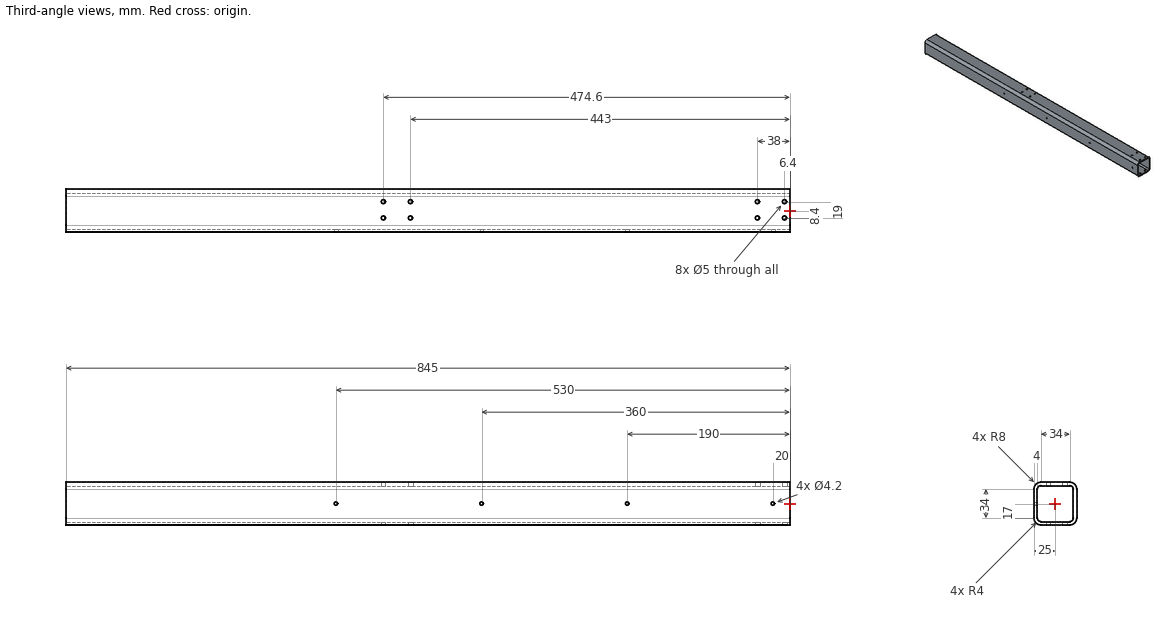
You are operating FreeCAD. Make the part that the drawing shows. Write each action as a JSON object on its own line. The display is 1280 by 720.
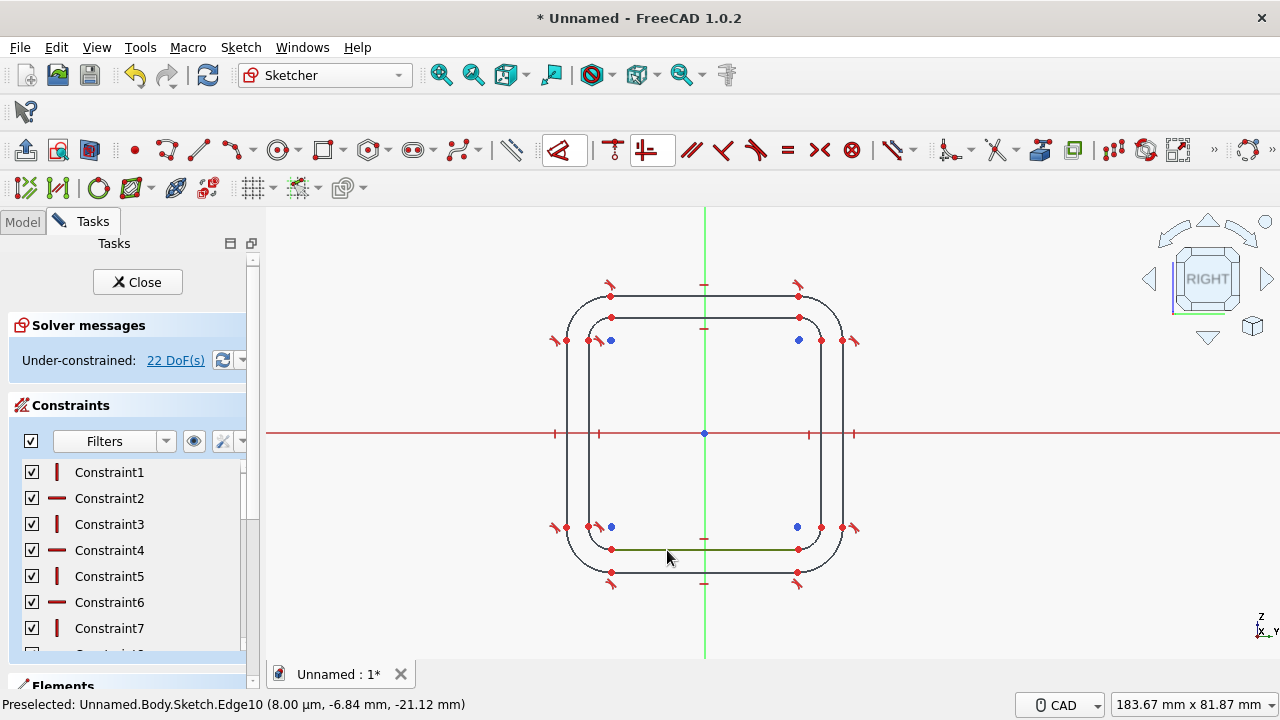
{"action": "scroll", "coordinate": [591, 537], "scroll_direction": "up", "scroll_amount": 2}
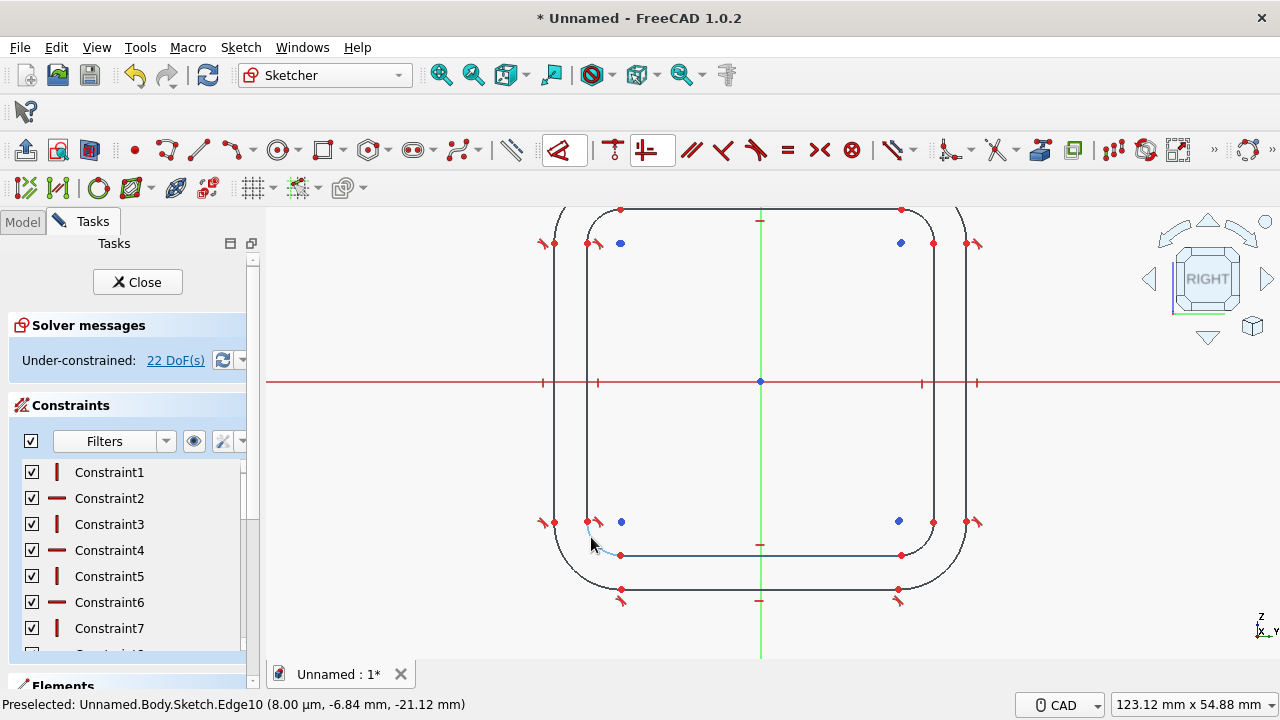
{"action": "left_click", "coordinate": [591, 537]}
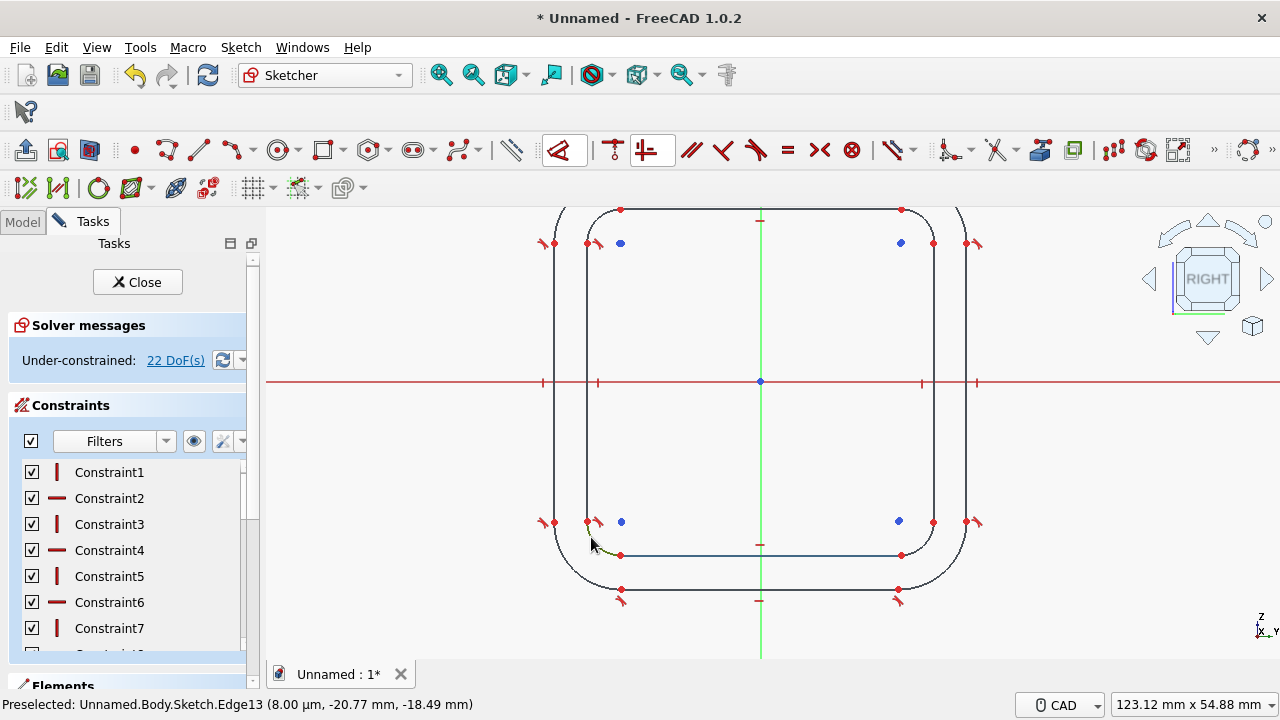
{"action": "left_click", "coordinate": [756, 150]}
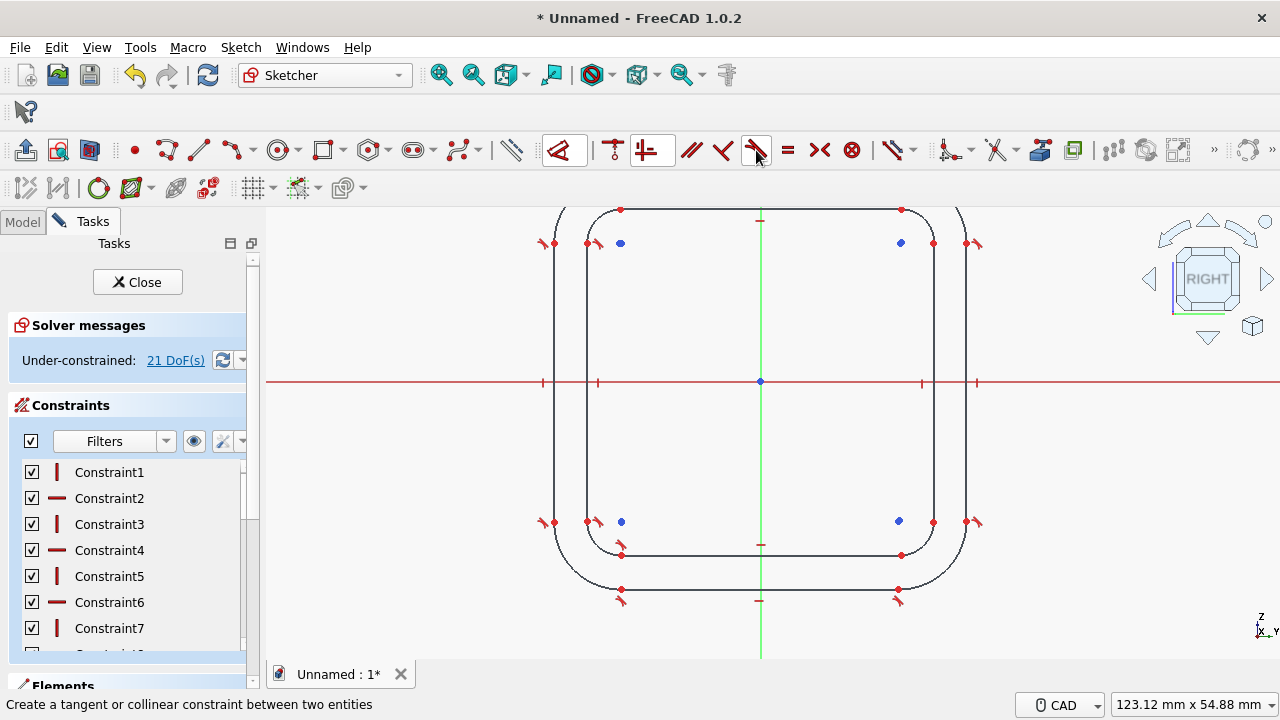
{"action": "left_click", "coordinate": [705, 556]}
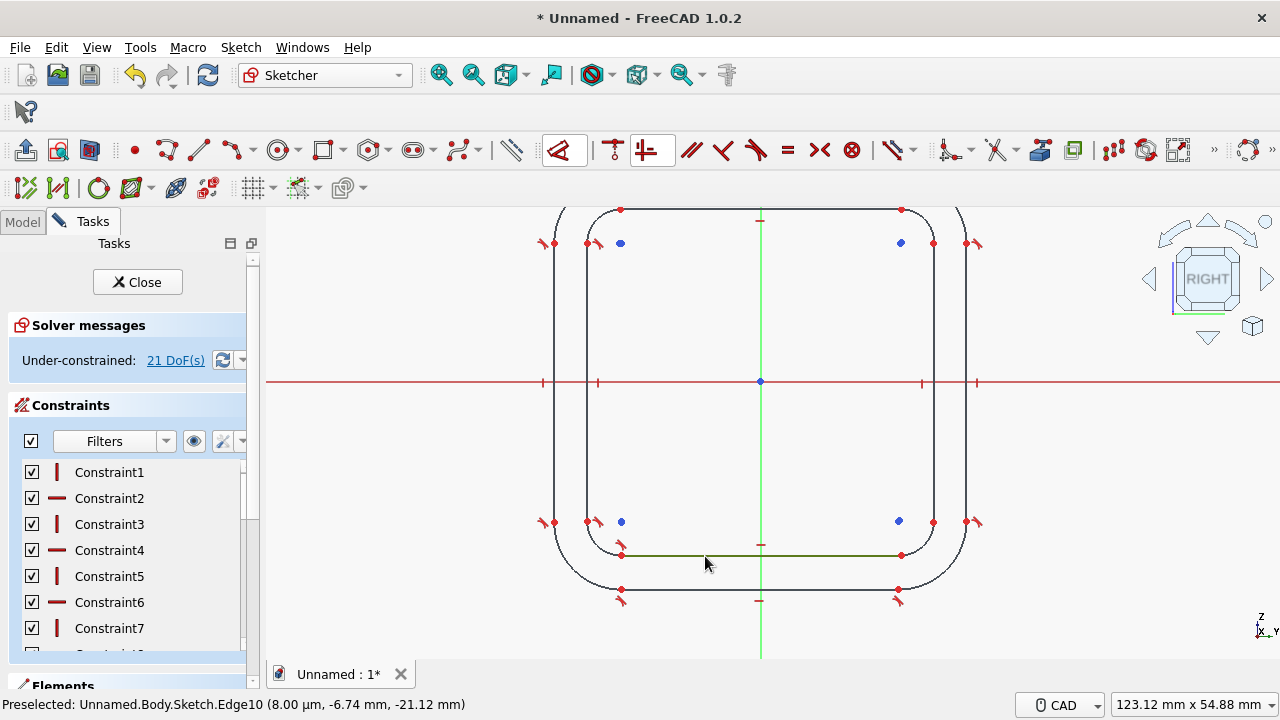
{"action": "left_click", "coordinate": [916, 551]}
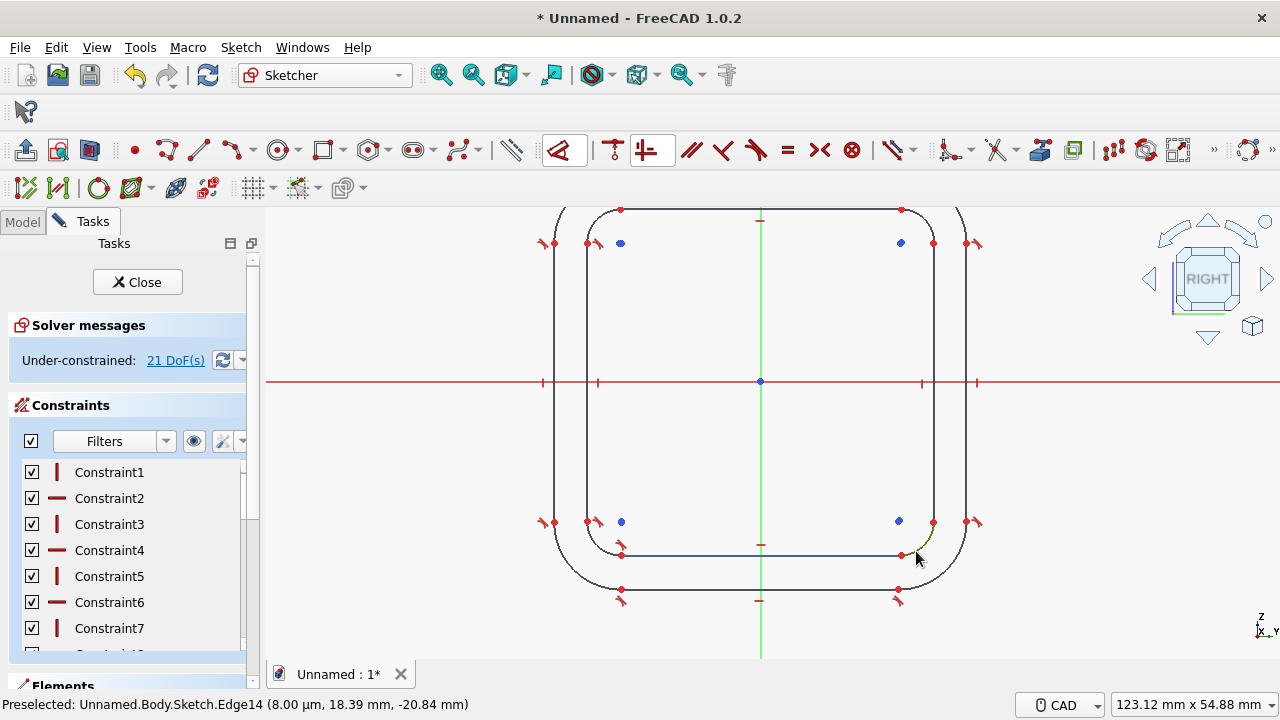
{"action": "left_click", "coordinate": [756, 150]}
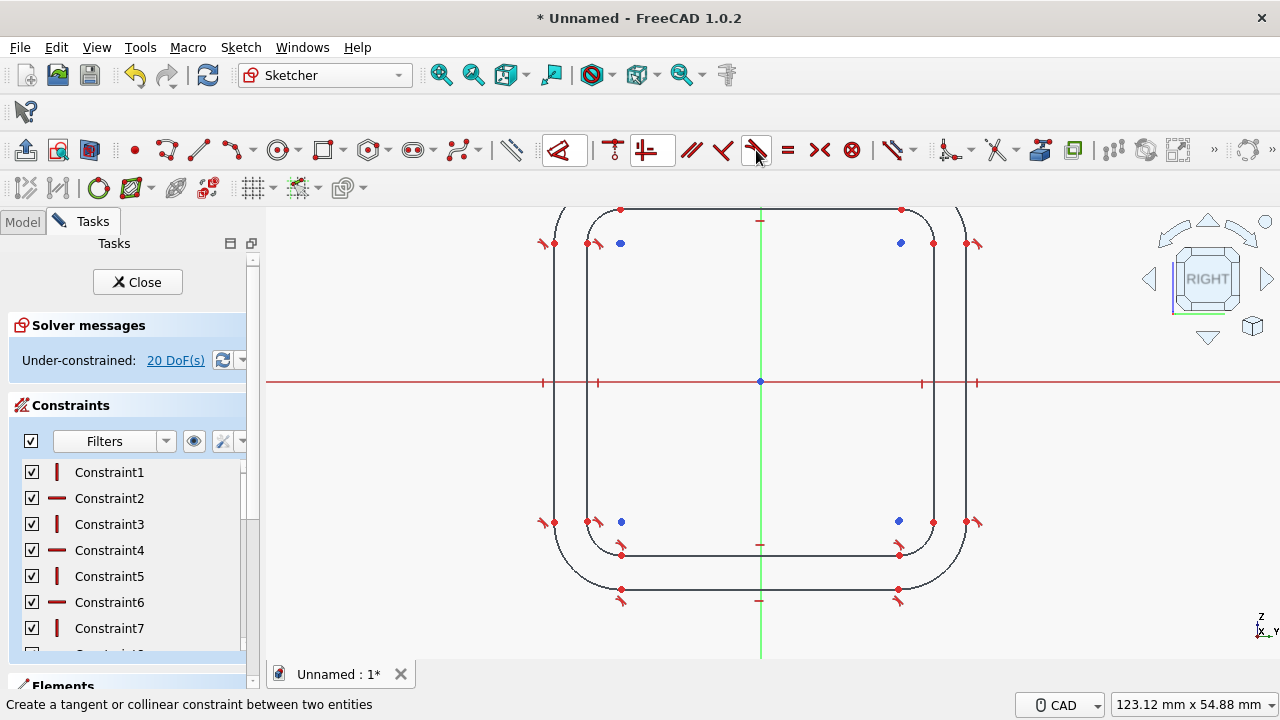
{"action": "left_click", "coordinate": [934, 439]}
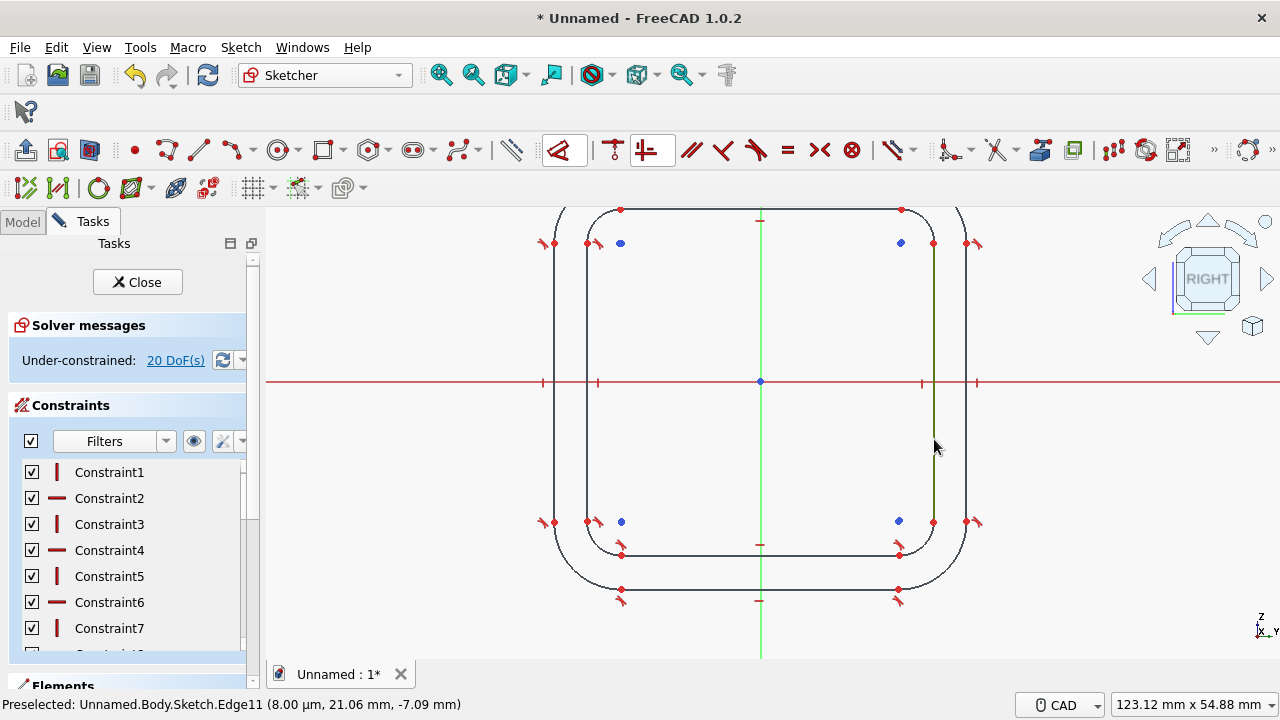
{"action": "left_click", "coordinate": [915, 552]}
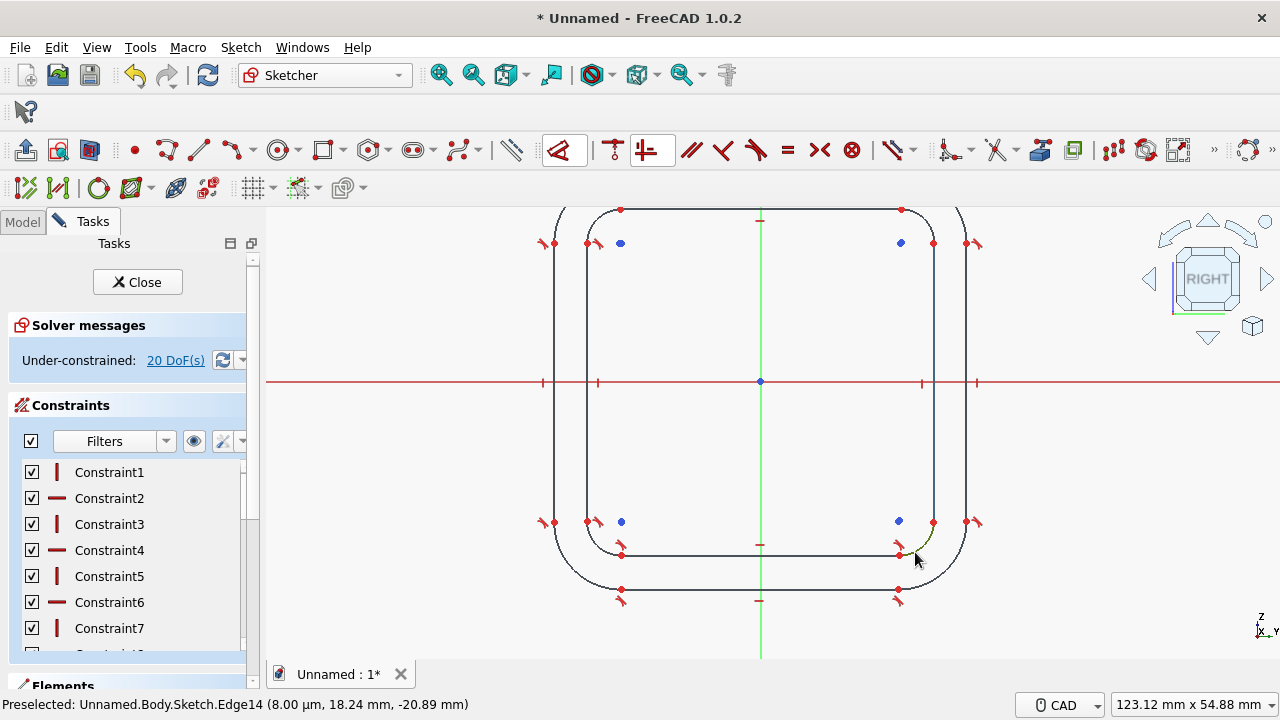
{"action": "left_click", "coordinate": [756, 150]}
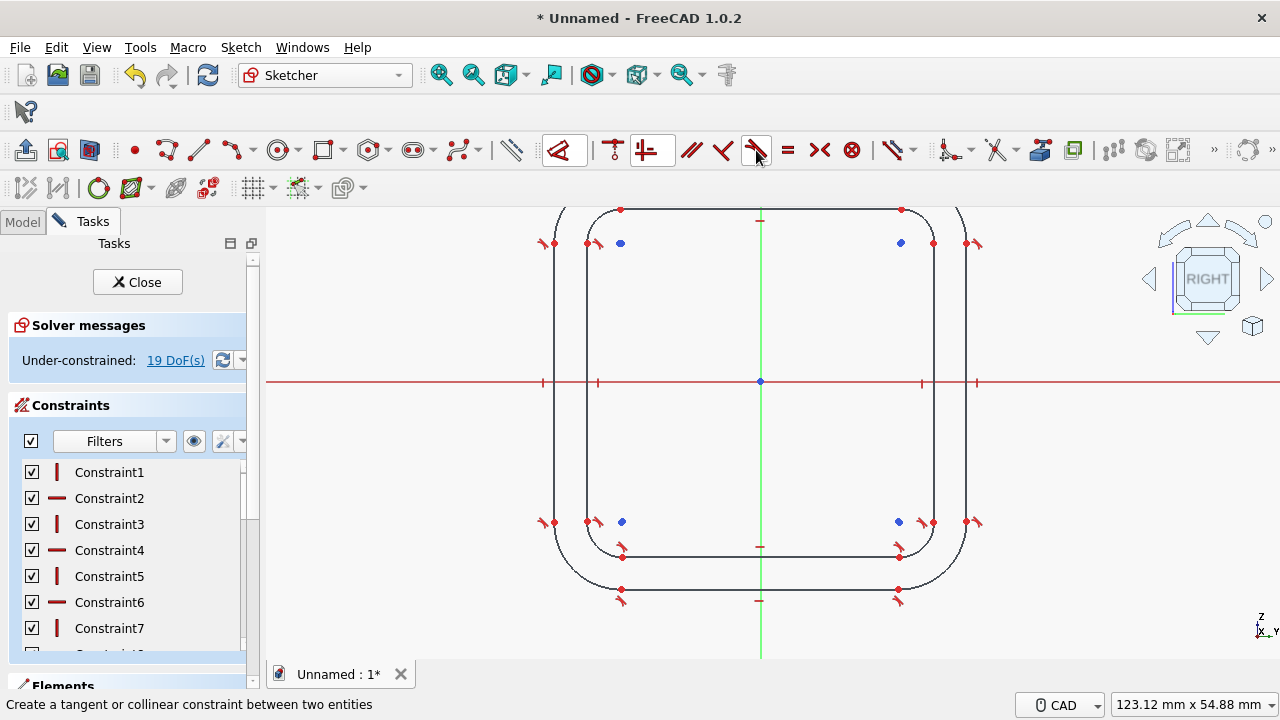
{"action": "left_click", "coordinate": [934, 439]}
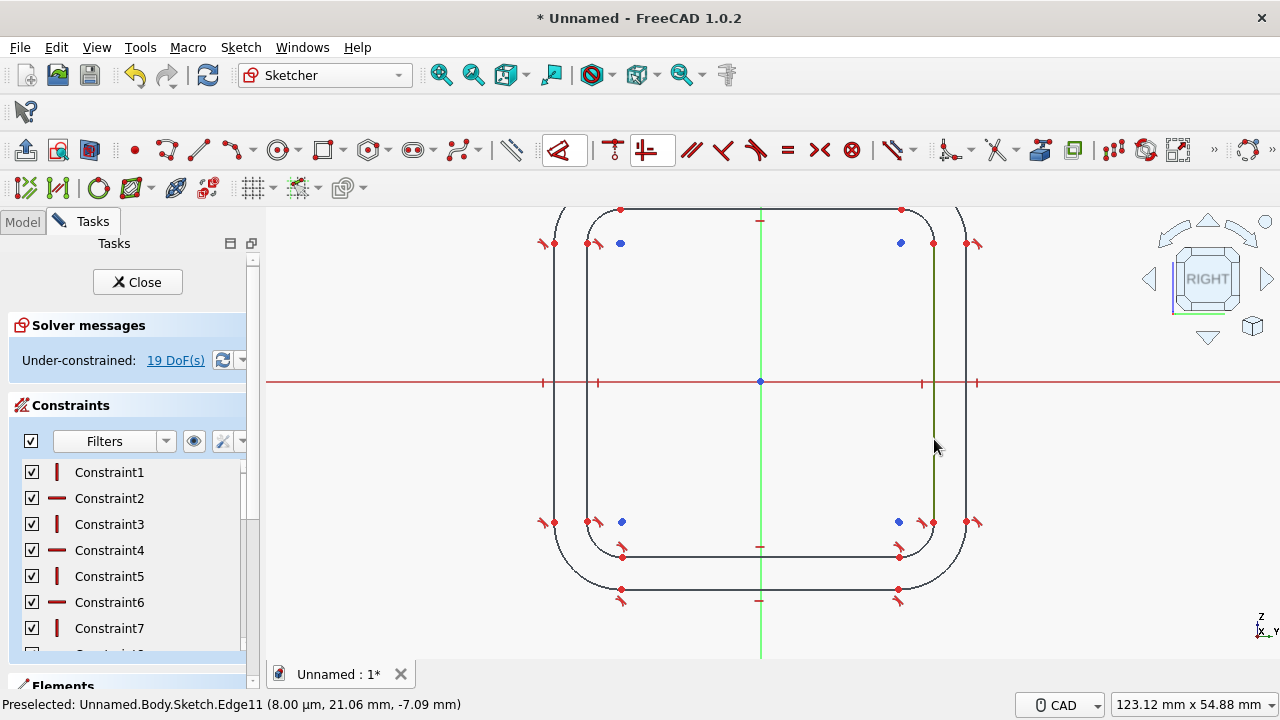
{"action": "scroll", "coordinate": [591, 538], "scroll_direction": "down", "scroll_amount": 2}